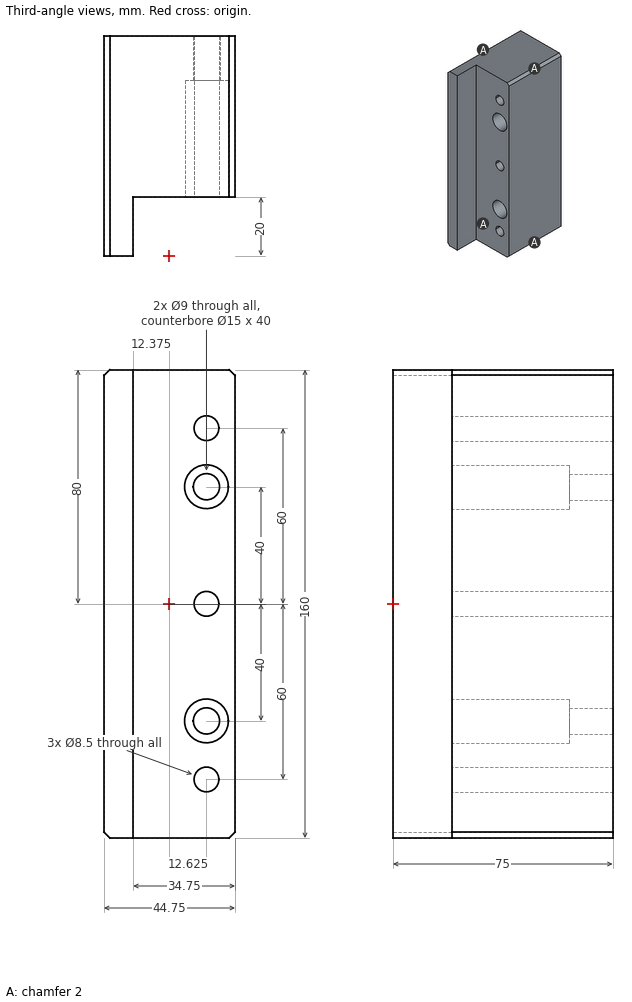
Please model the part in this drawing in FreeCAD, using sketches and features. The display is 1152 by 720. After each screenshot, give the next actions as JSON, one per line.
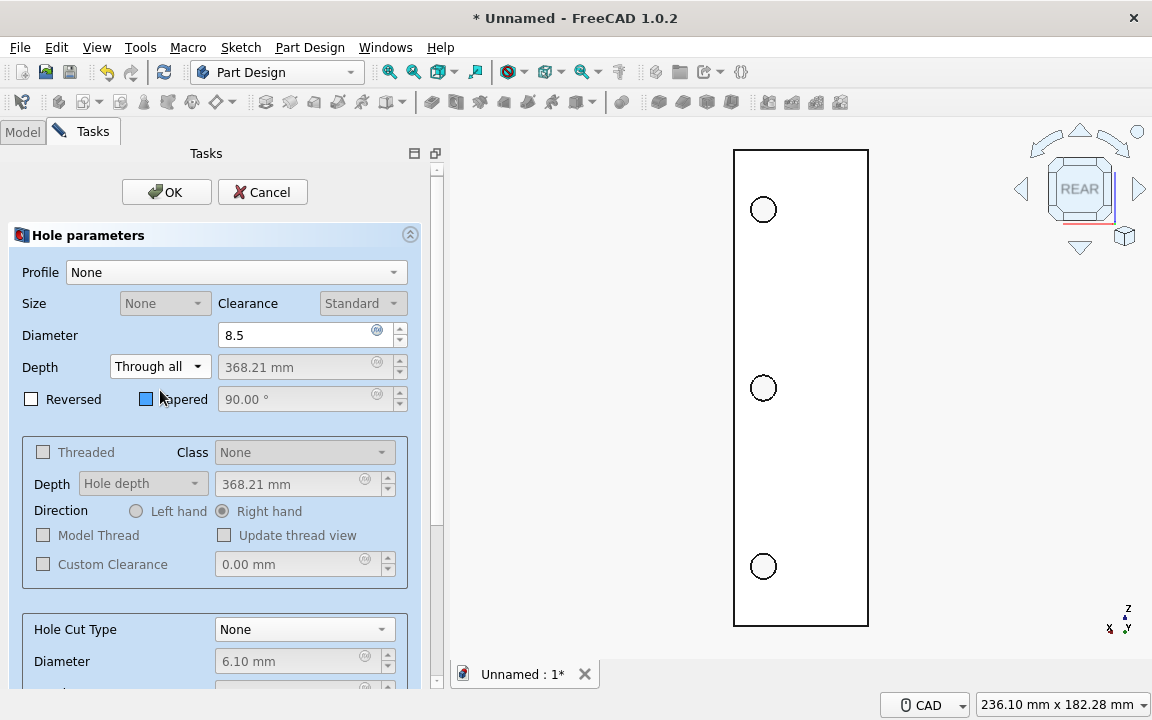
{"action": "left_click", "coordinate": [167, 192]}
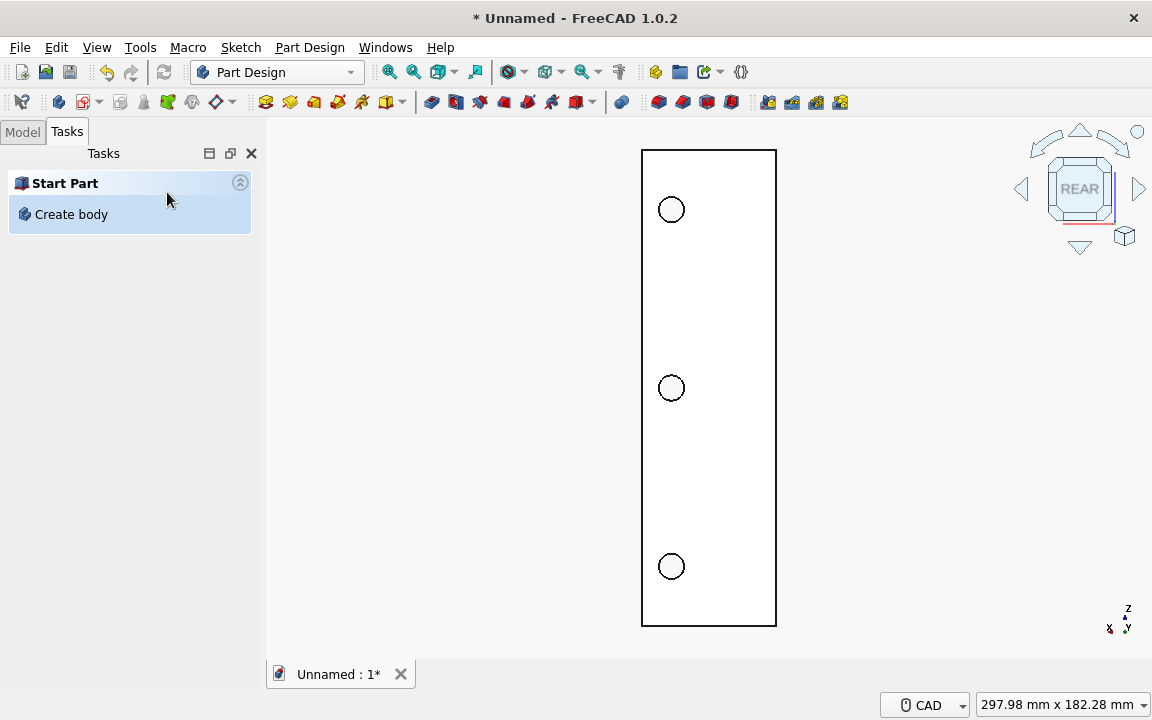
{"action": "key", "text": "0"}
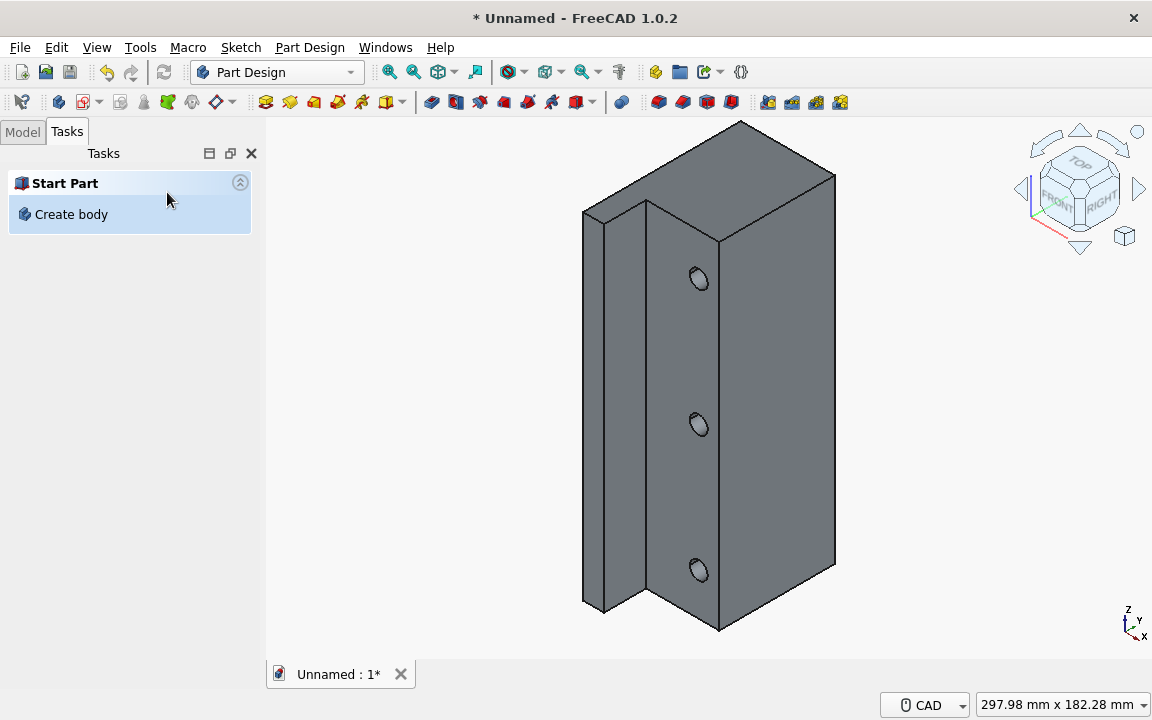
{"action": "left_click", "coordinate": [777, 208]}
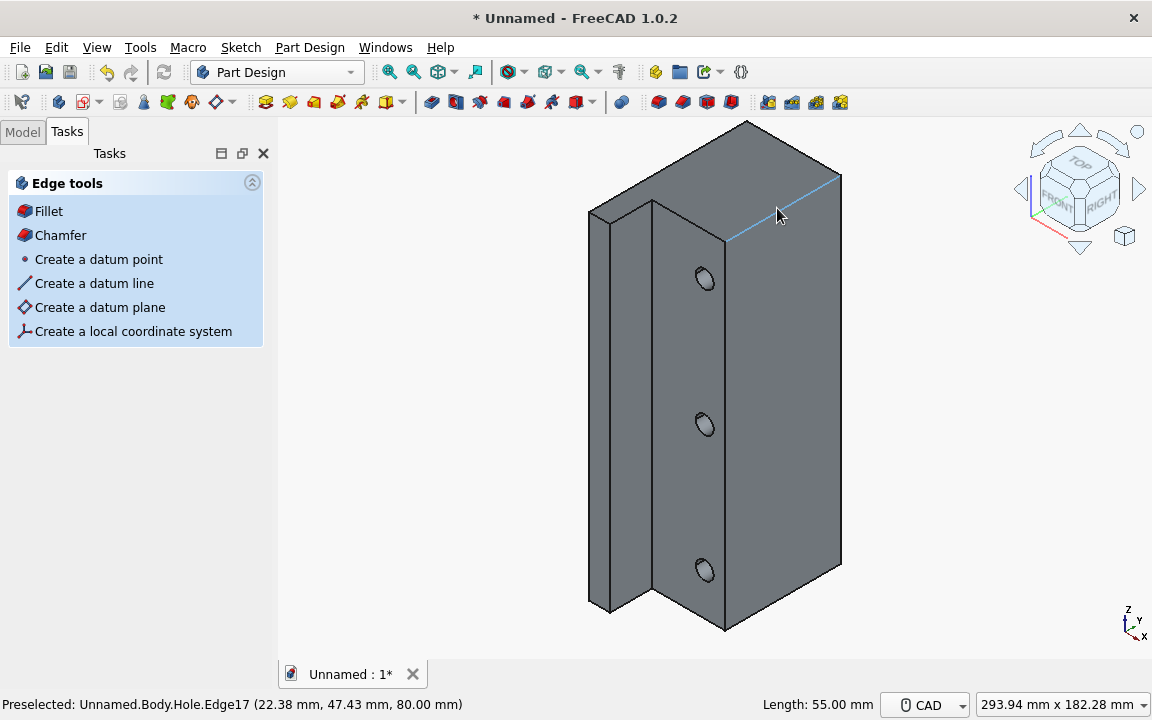
{"action": "key", "text": "2"}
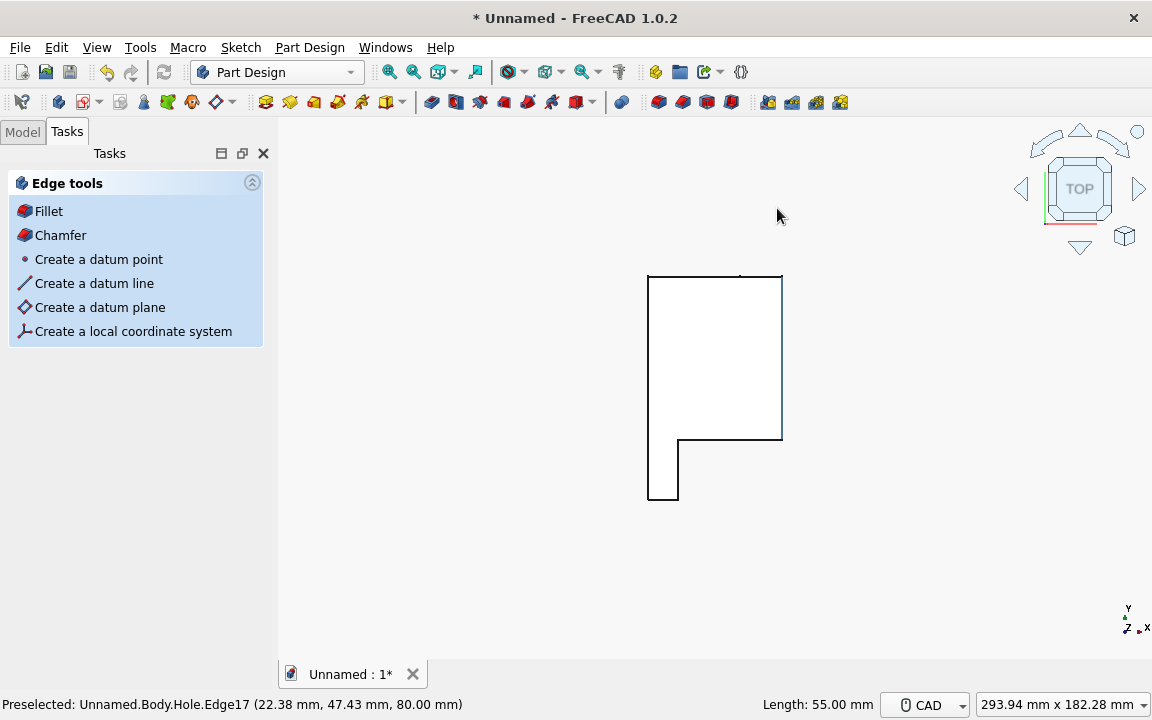
{"action": "left_click", "coordinate": [390, 72]}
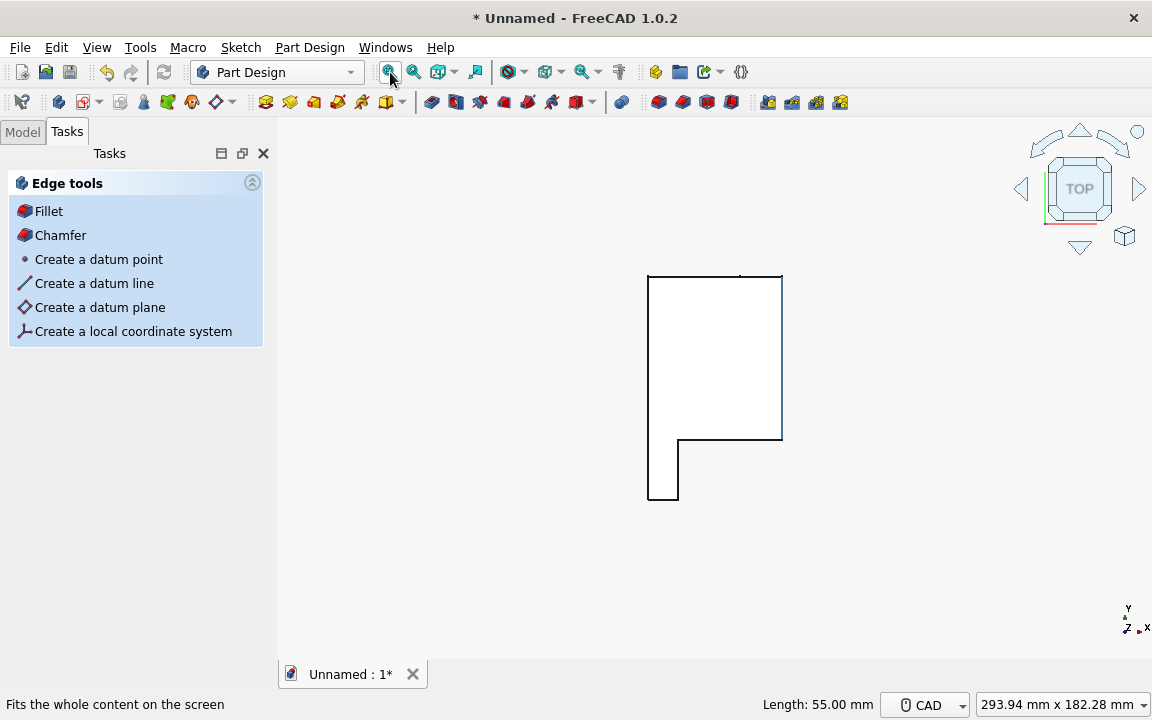
{"action": "left_click", "coordinate": [648, 387], "text": "ctrl"}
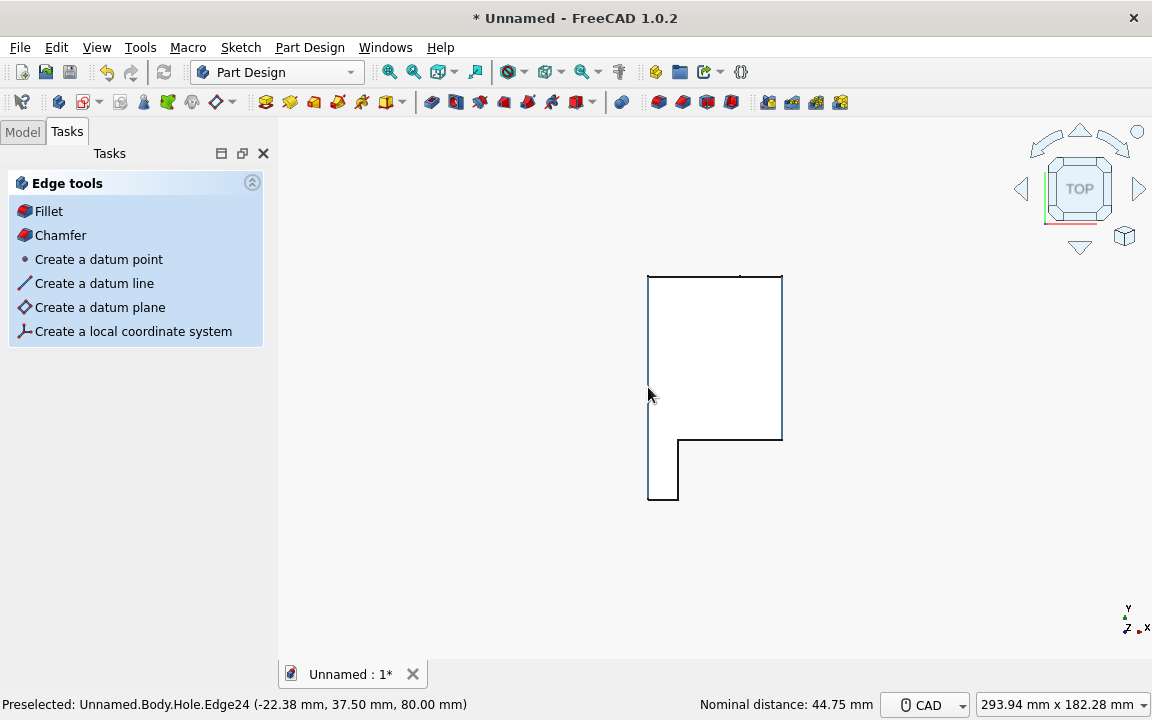
{"action": "key", "text": "1"}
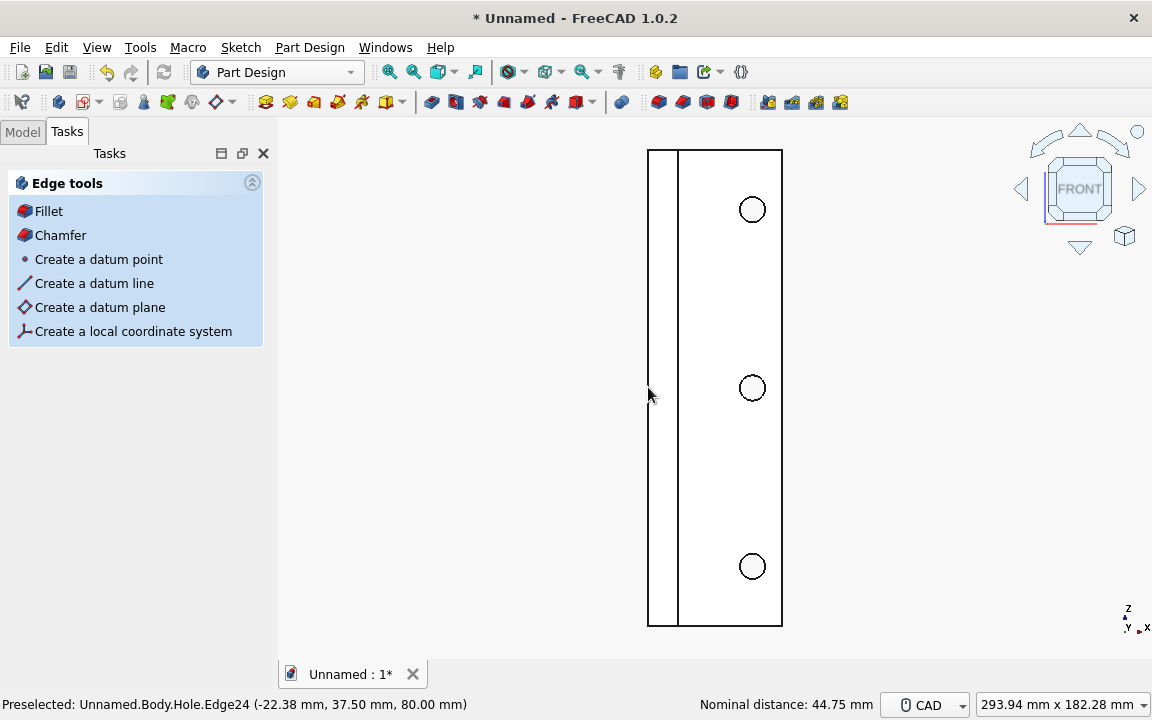
{"action": "key", "text": "3"}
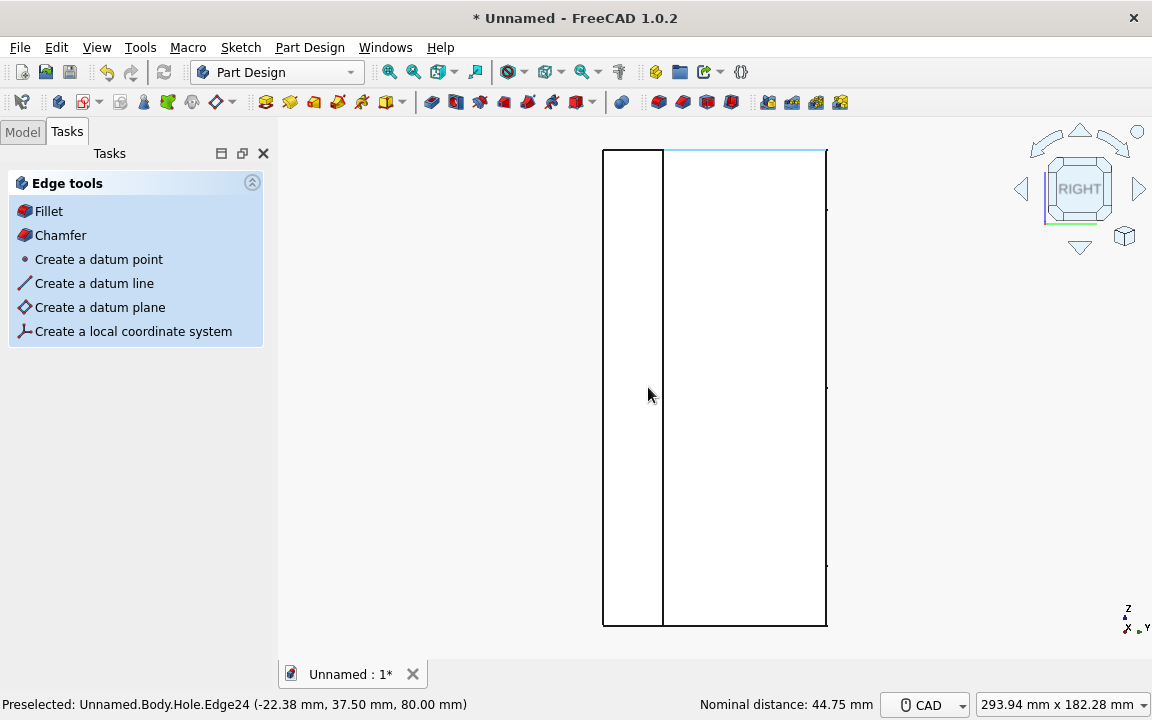
{"action": "left_click", "coordinate": [745, 625], "text": "ctrl"}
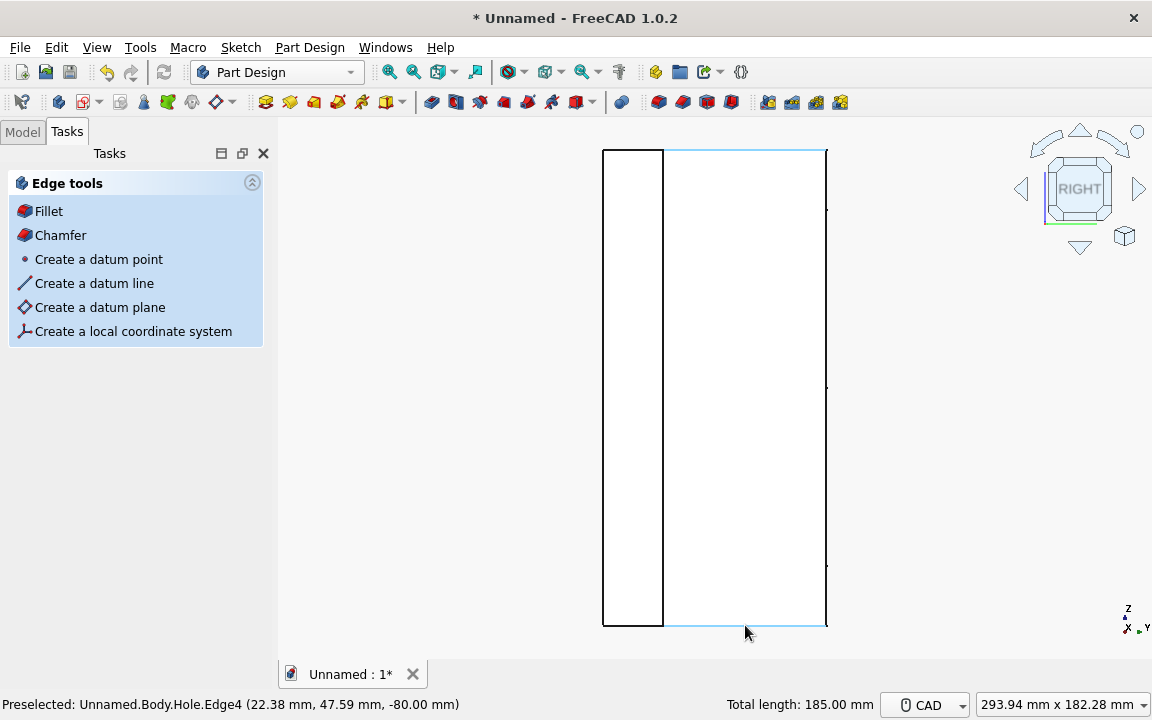
{"action": "key", "text": "5"}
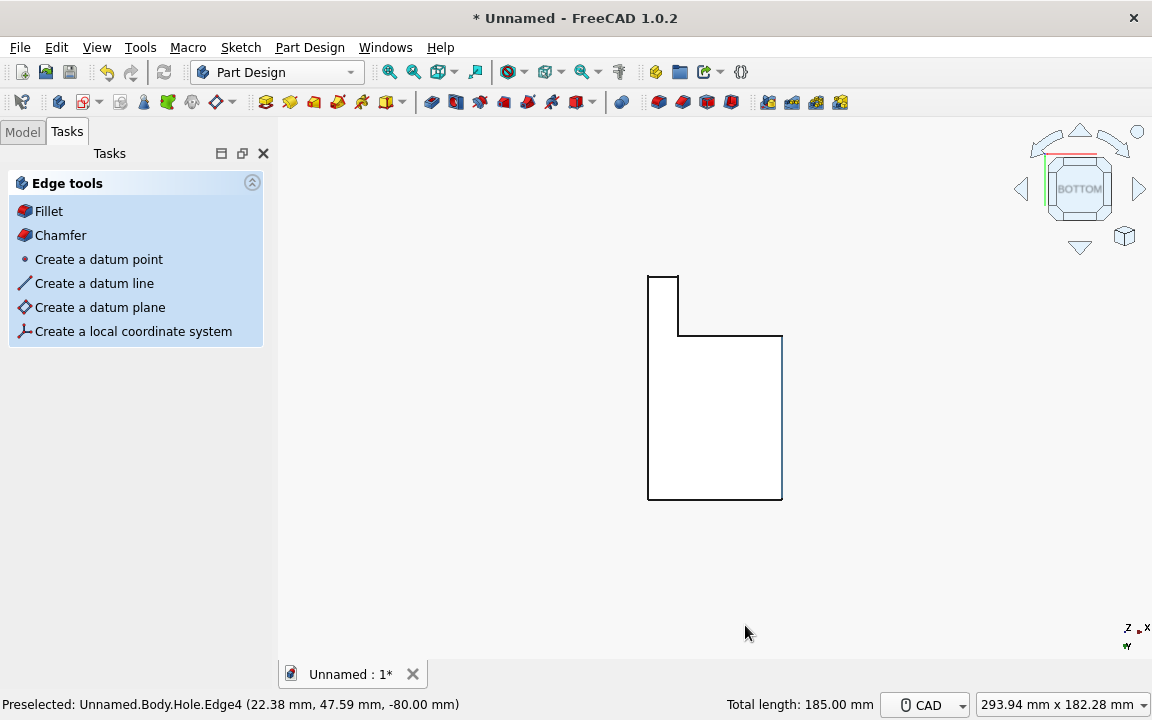
{"action": "left_click", "coordinate": [390, 72]}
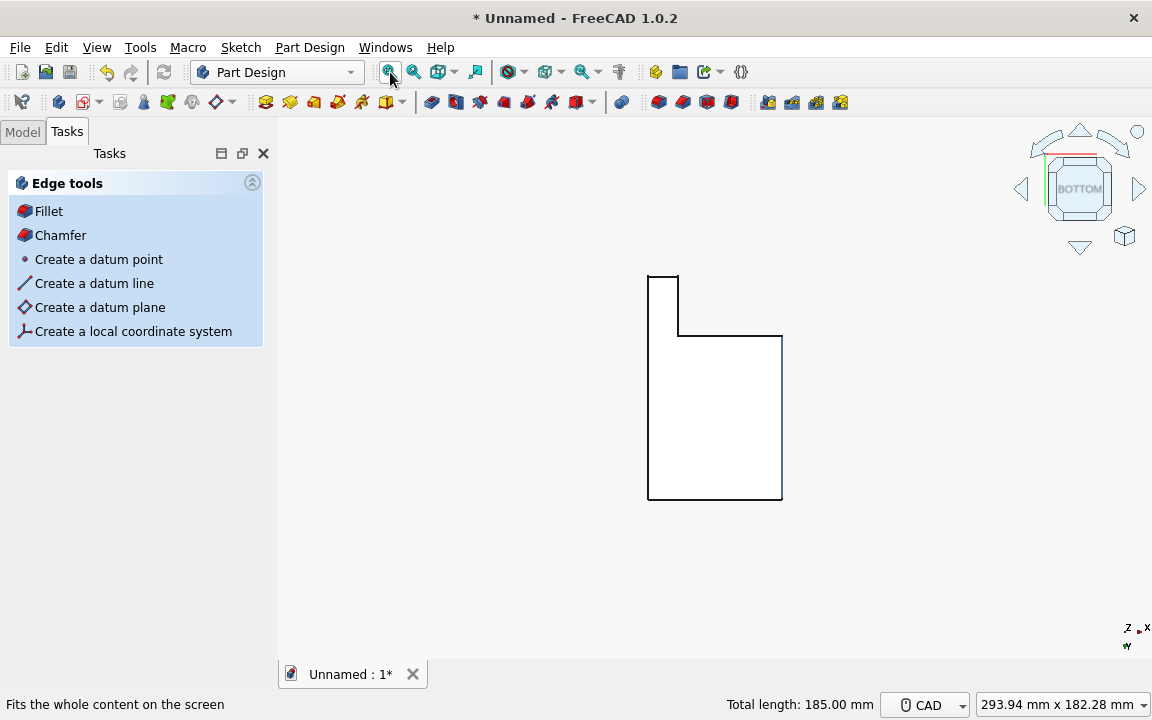
{"action": "left_click", "coordinate": [648, 387], "text": "ctrl"}